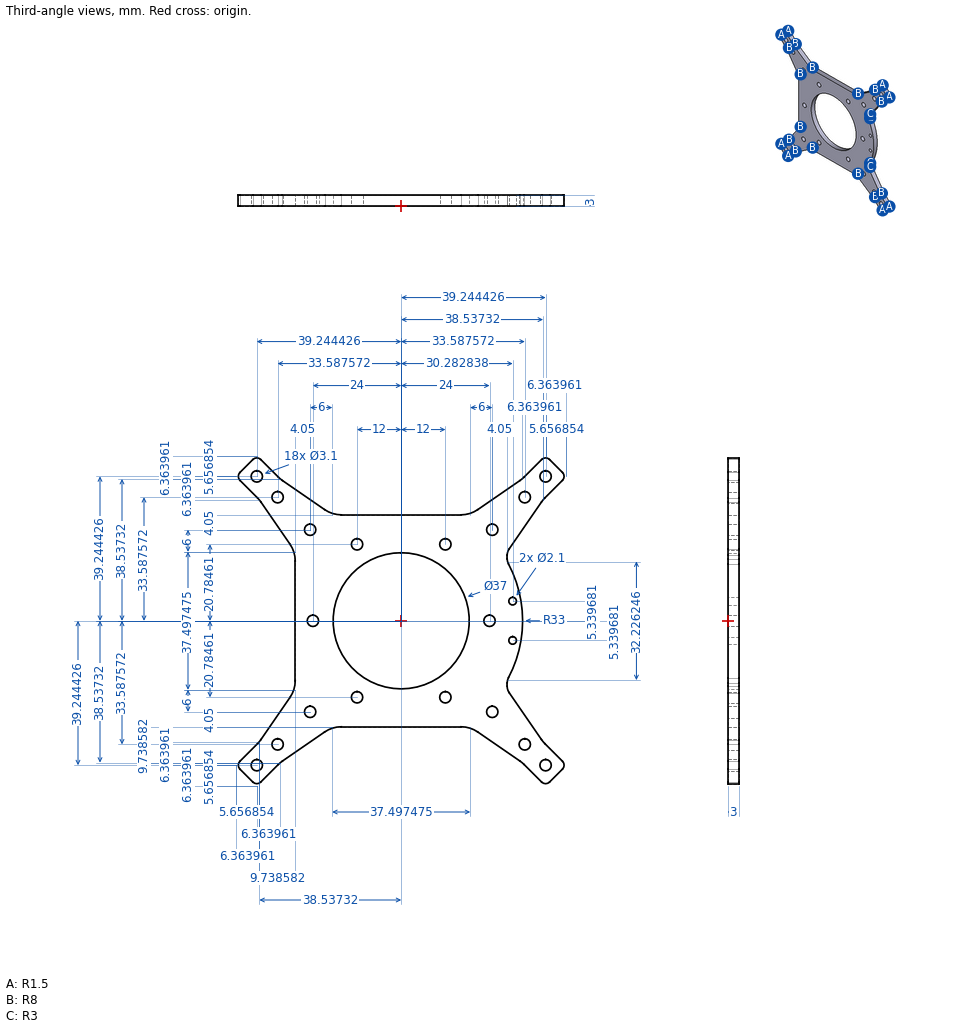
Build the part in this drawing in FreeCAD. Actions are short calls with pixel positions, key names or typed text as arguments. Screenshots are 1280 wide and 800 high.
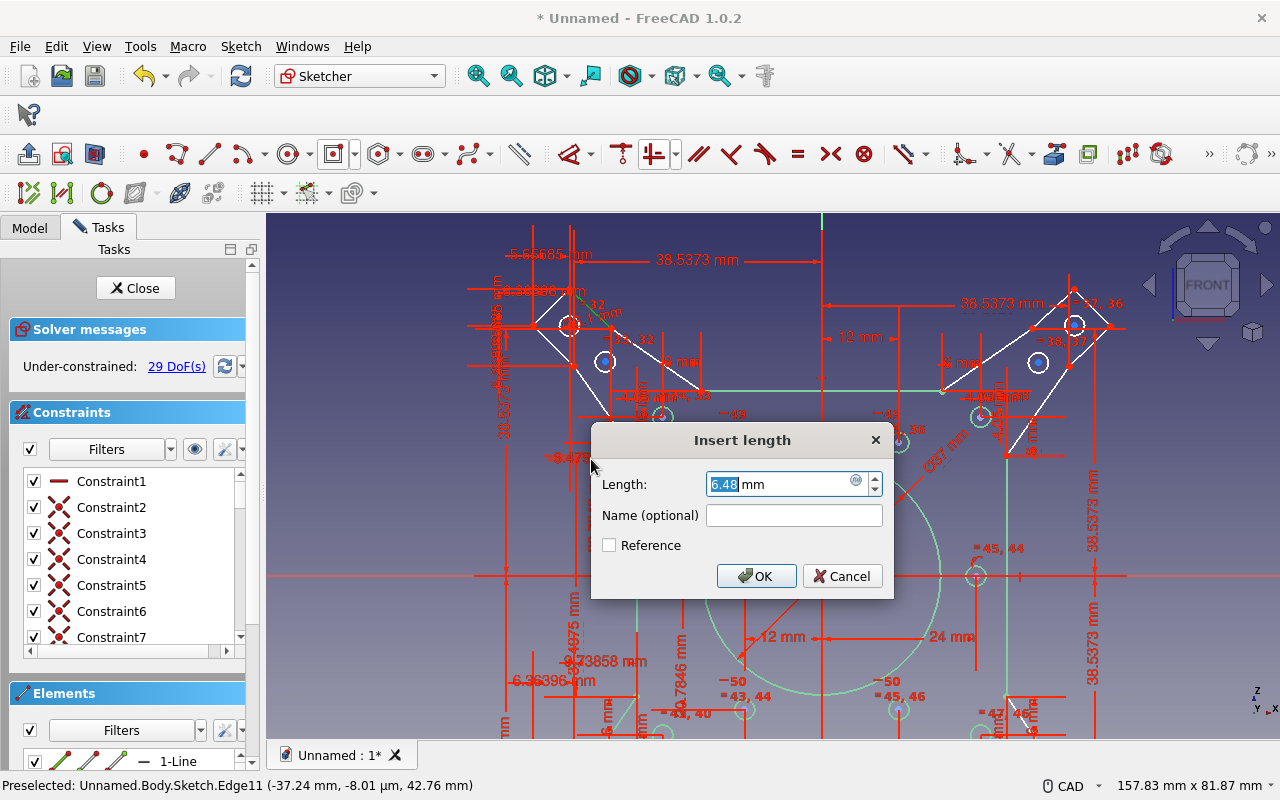
text(6.363961)
key(Return)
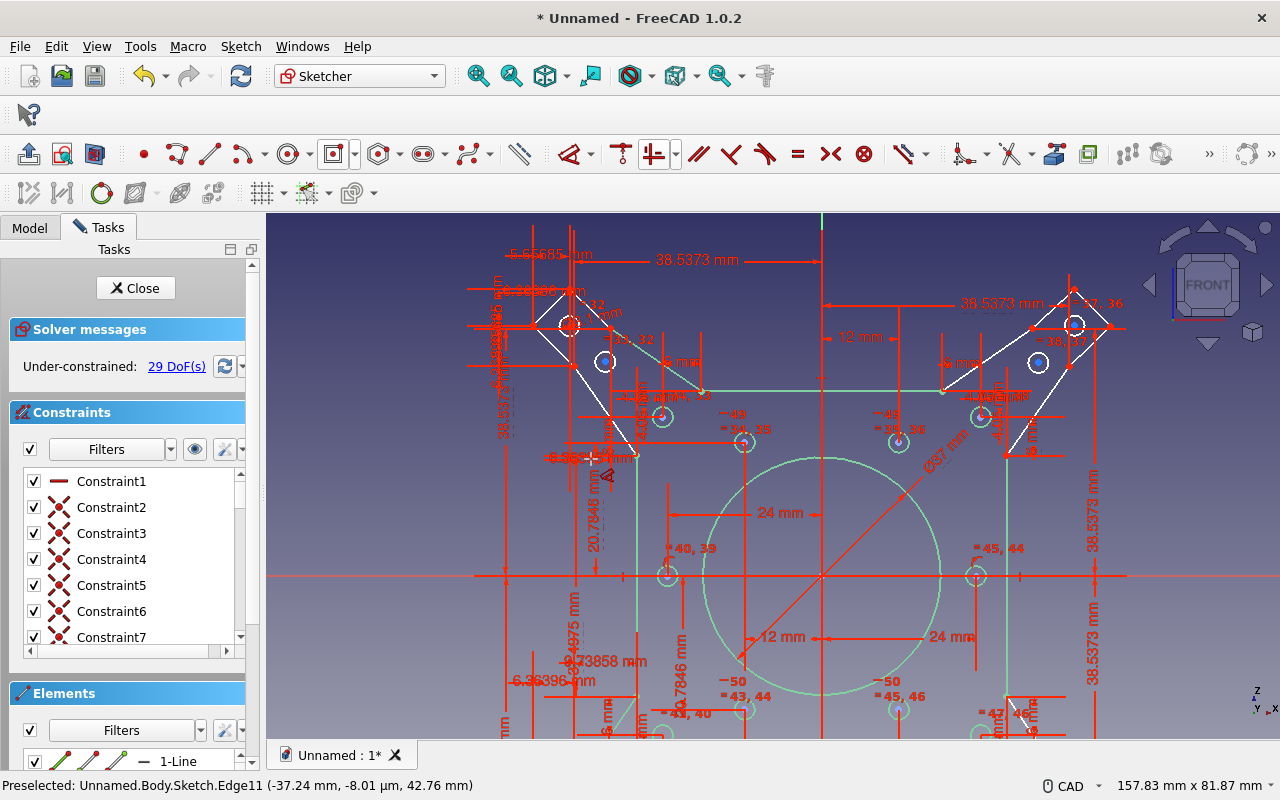
click(582, 301)
click(645, 300)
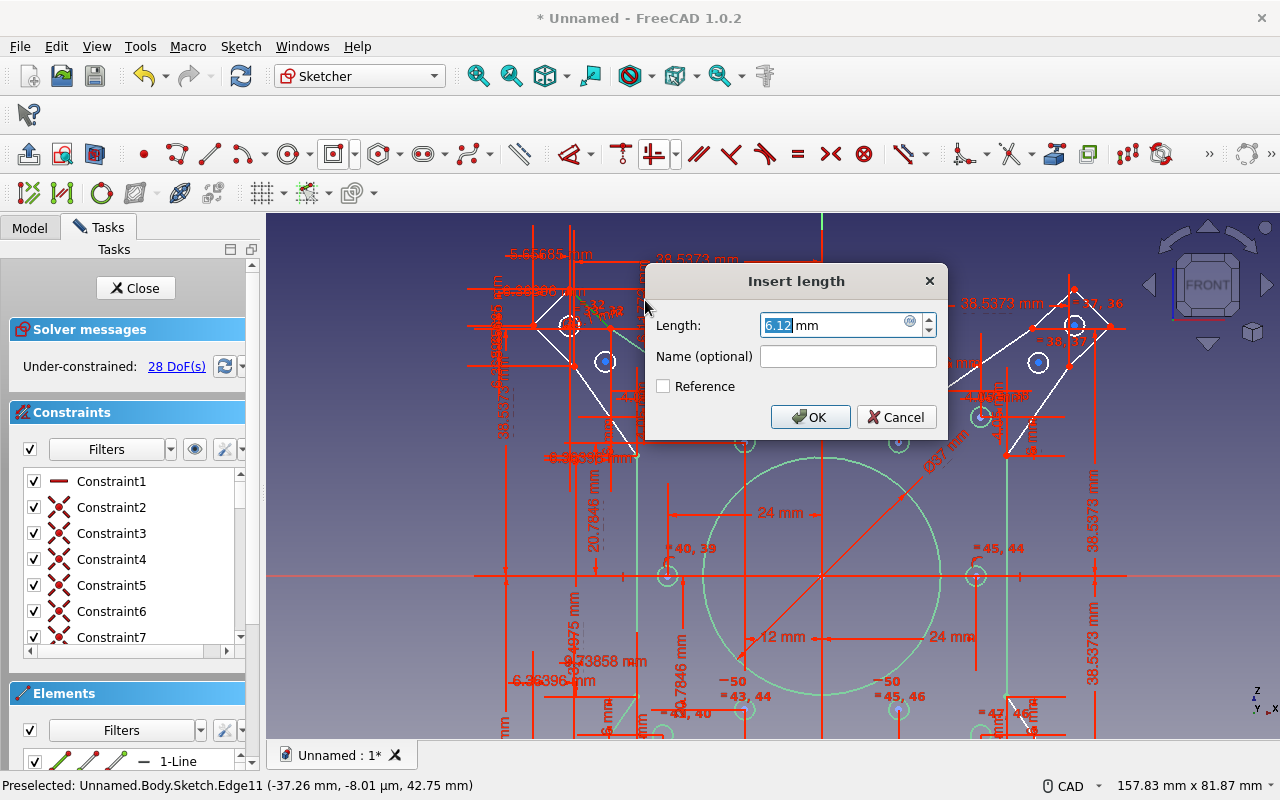
text(6.363961)
key(Return)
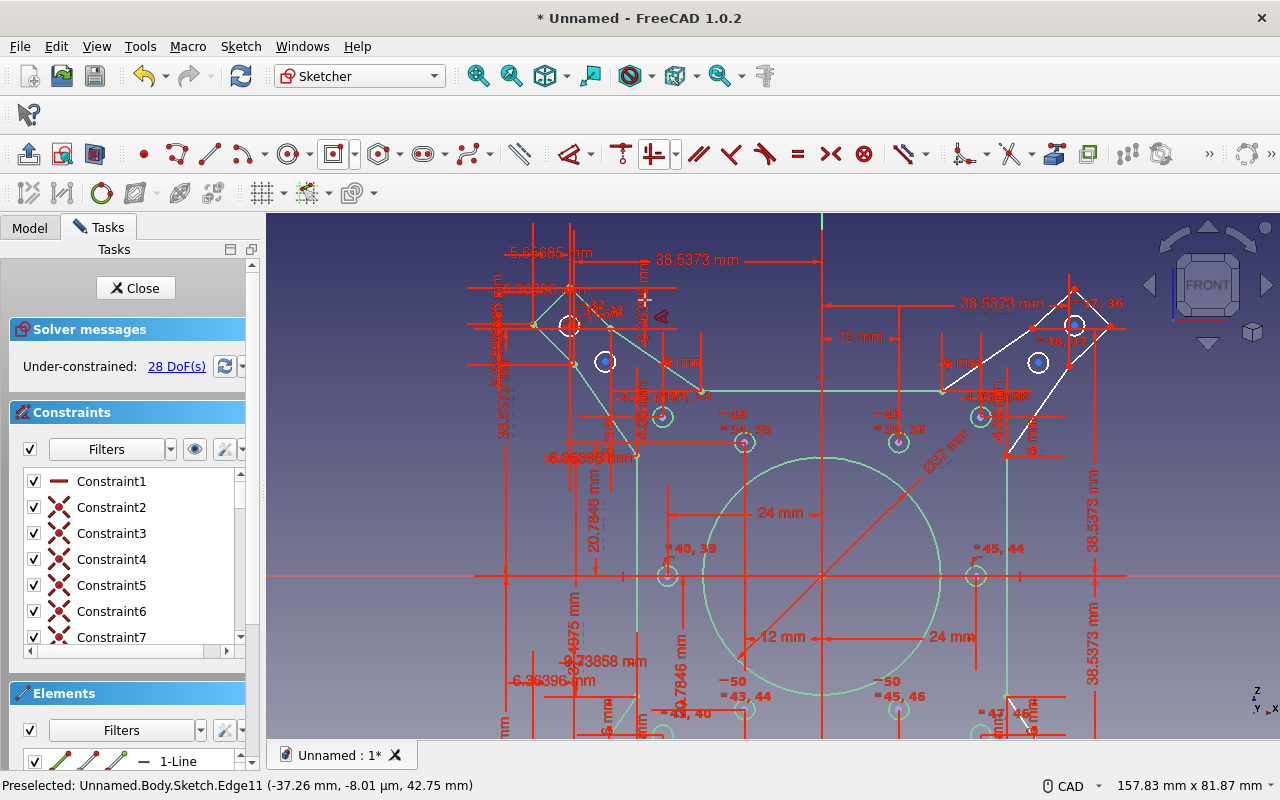
click(1045, 317)
click(1053, 256)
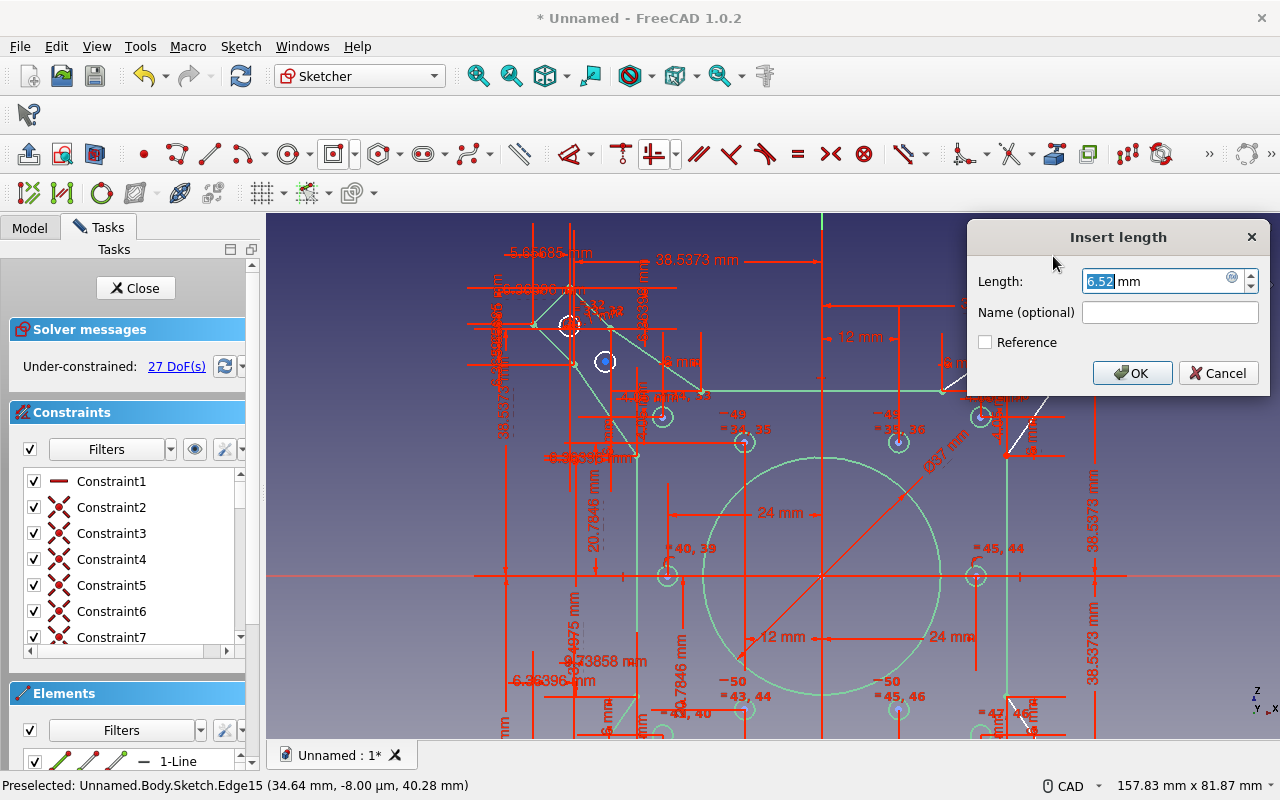
text(6.363961)
key(Return)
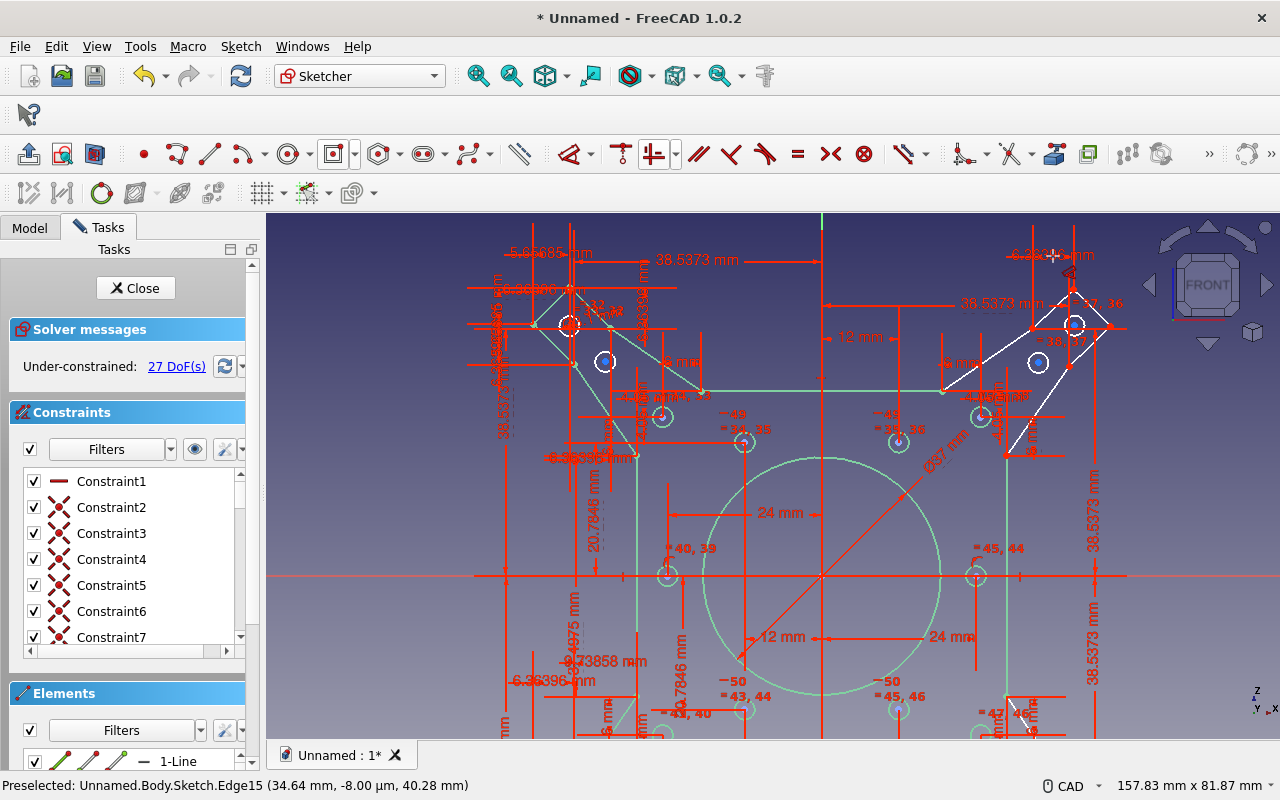
click(1045, 317)
click(1108, 300)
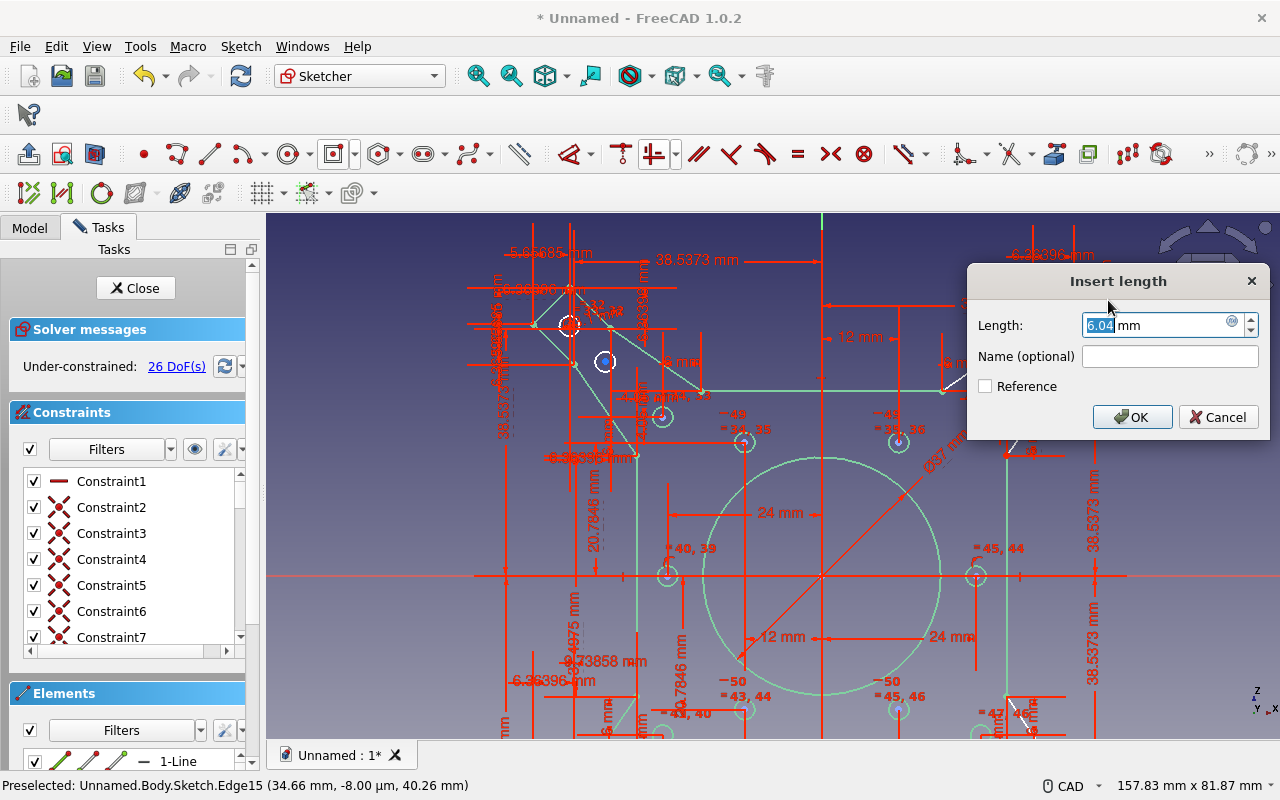
text(6.363961)
key(Return)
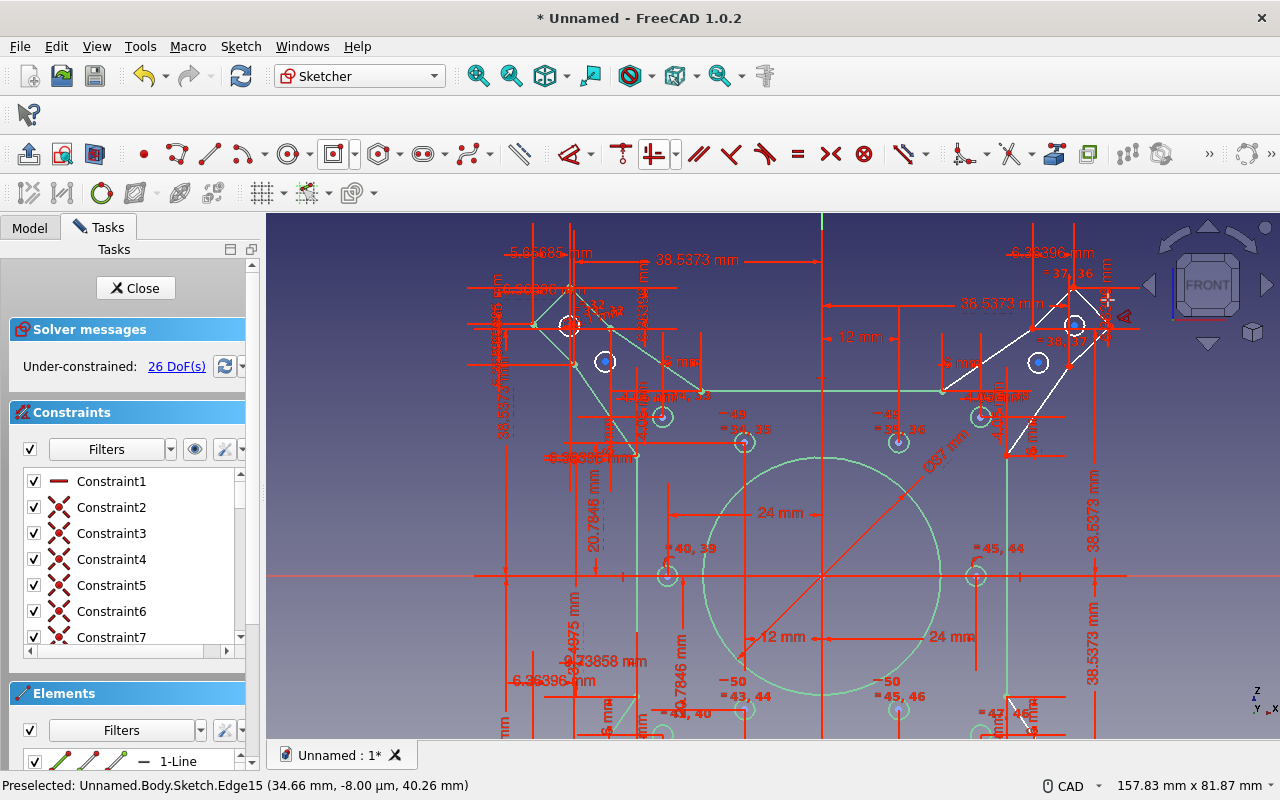
click(1085, 299)
click(1101, 360)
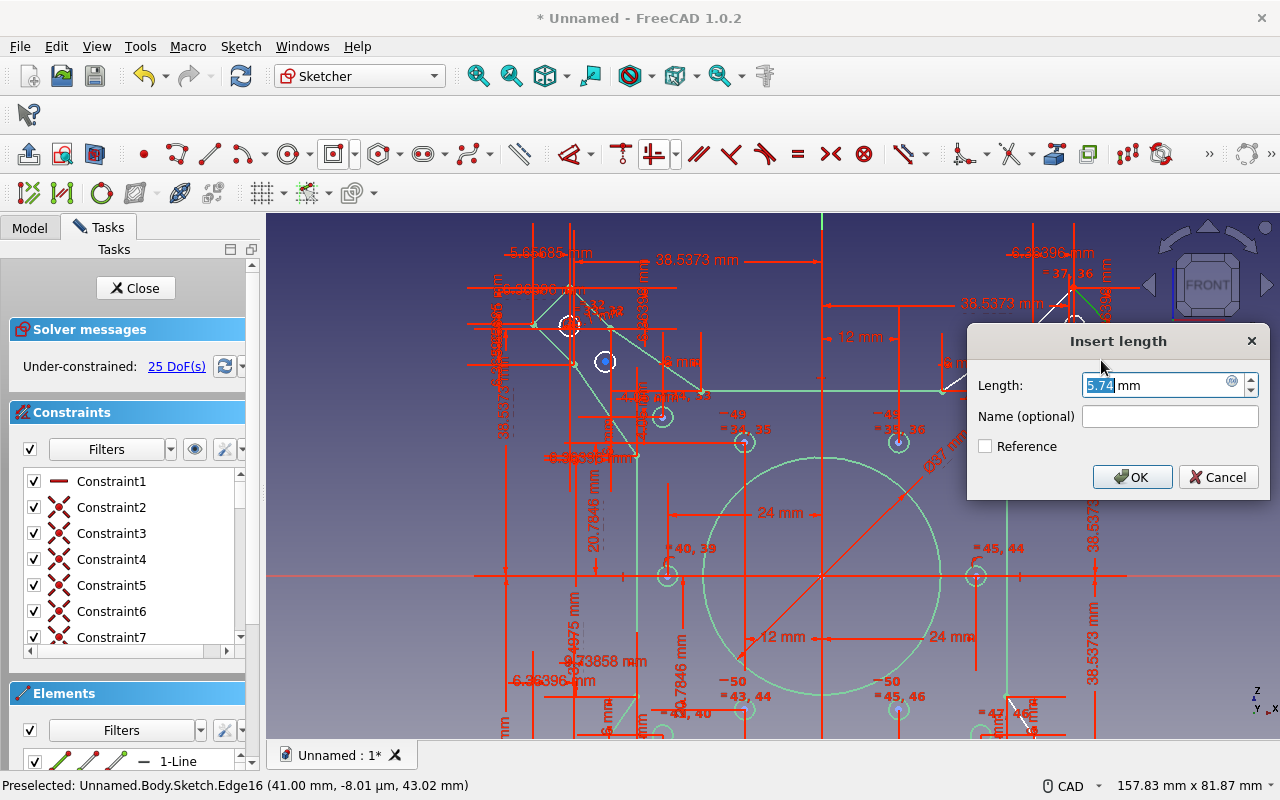
text(5.656854)
key(Return)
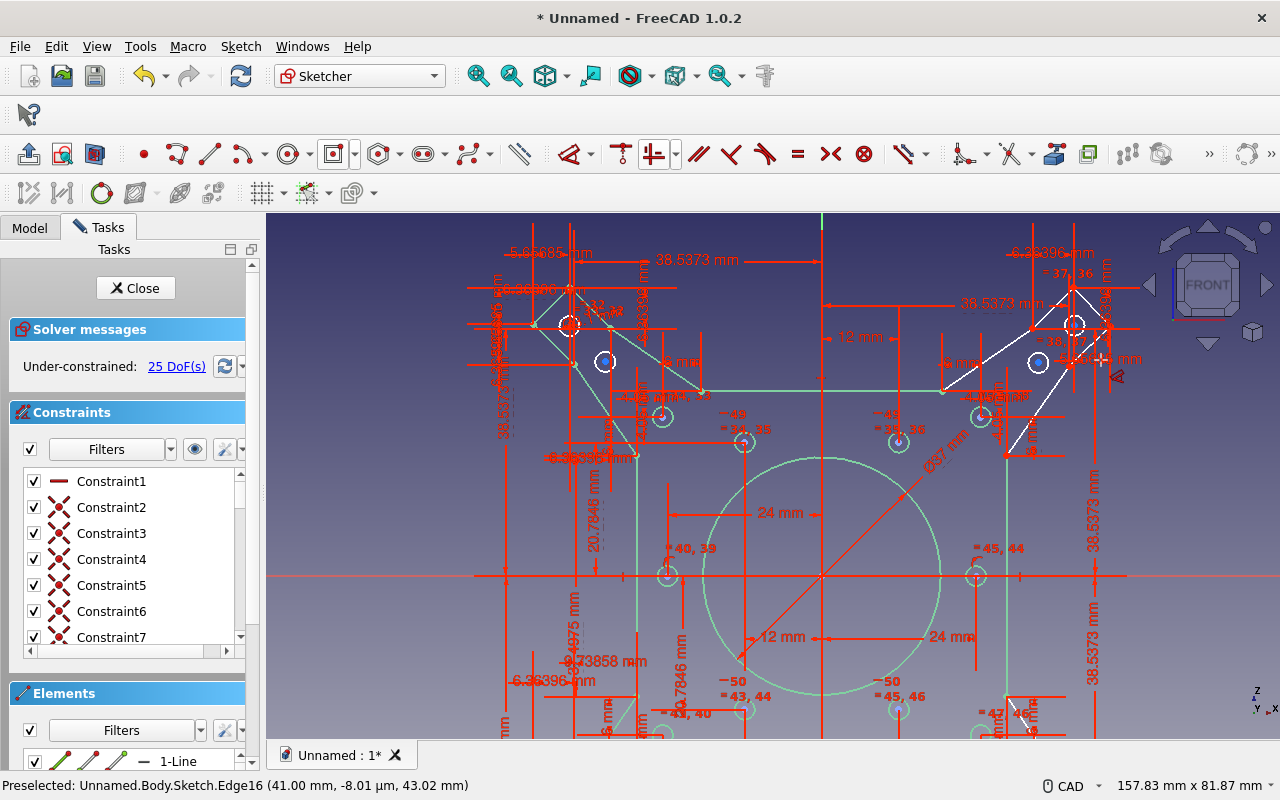
click(1085, 299)
click(920, 307)